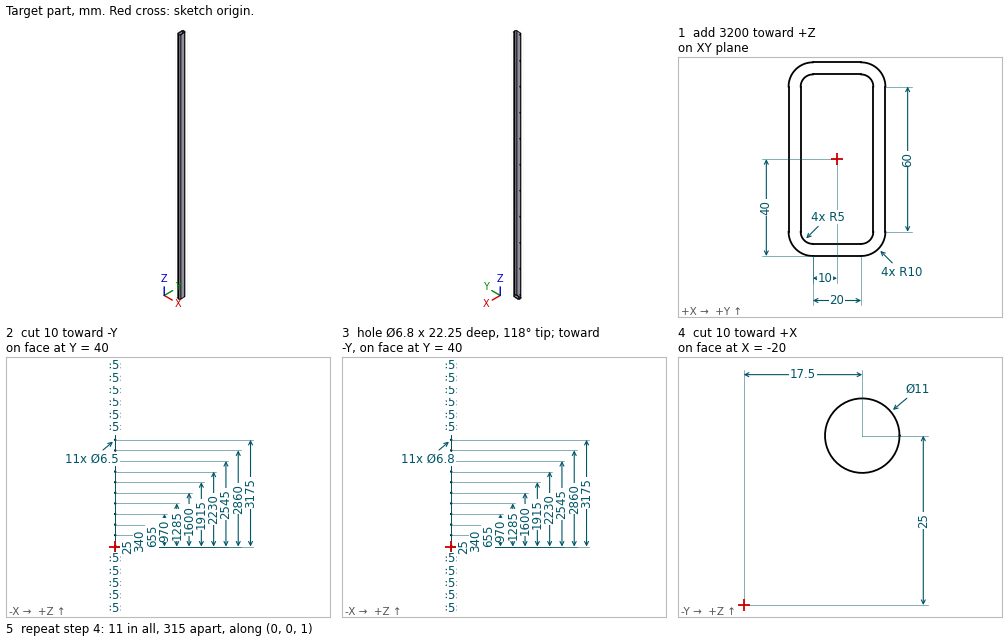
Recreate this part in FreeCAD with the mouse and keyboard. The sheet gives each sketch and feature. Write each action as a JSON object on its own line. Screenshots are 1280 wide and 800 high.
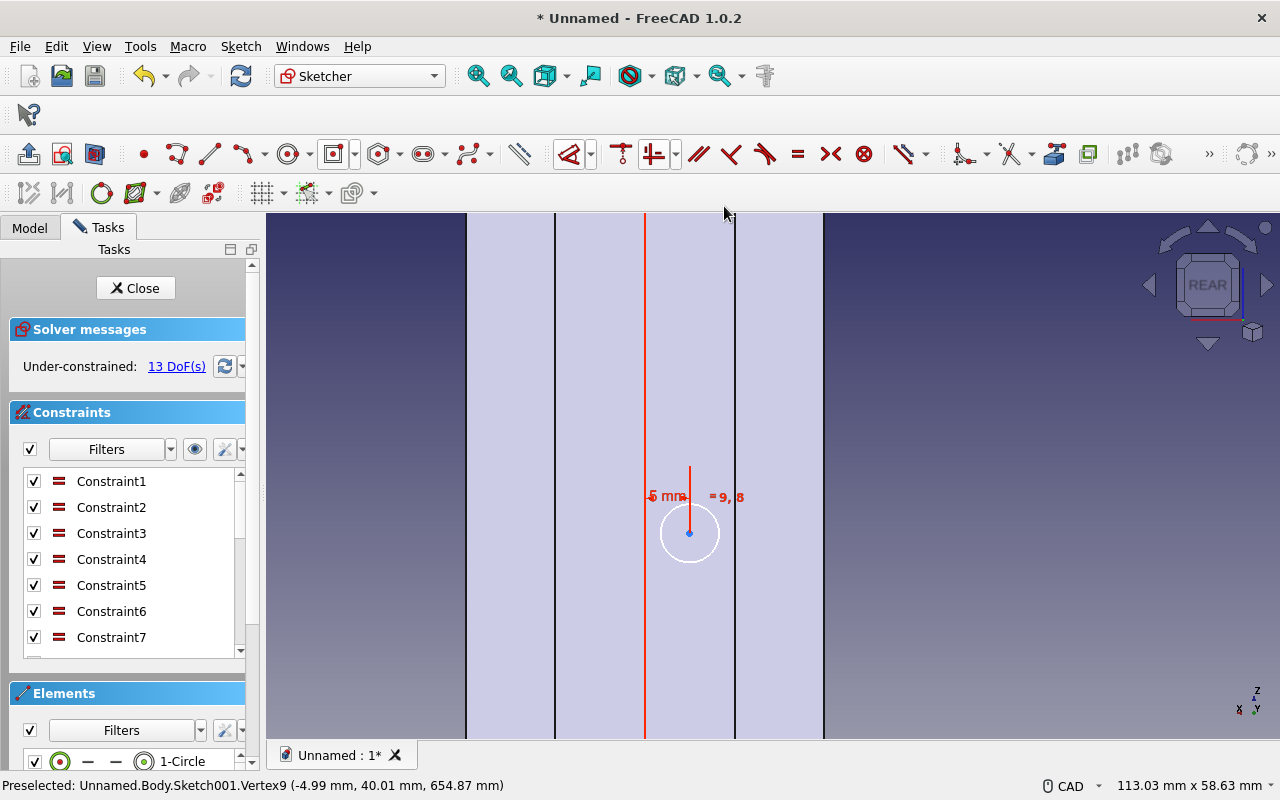
{"action": "scroll", "coordinate": [704, 476], "scroll_direction": "down", "scroll_amount": 15}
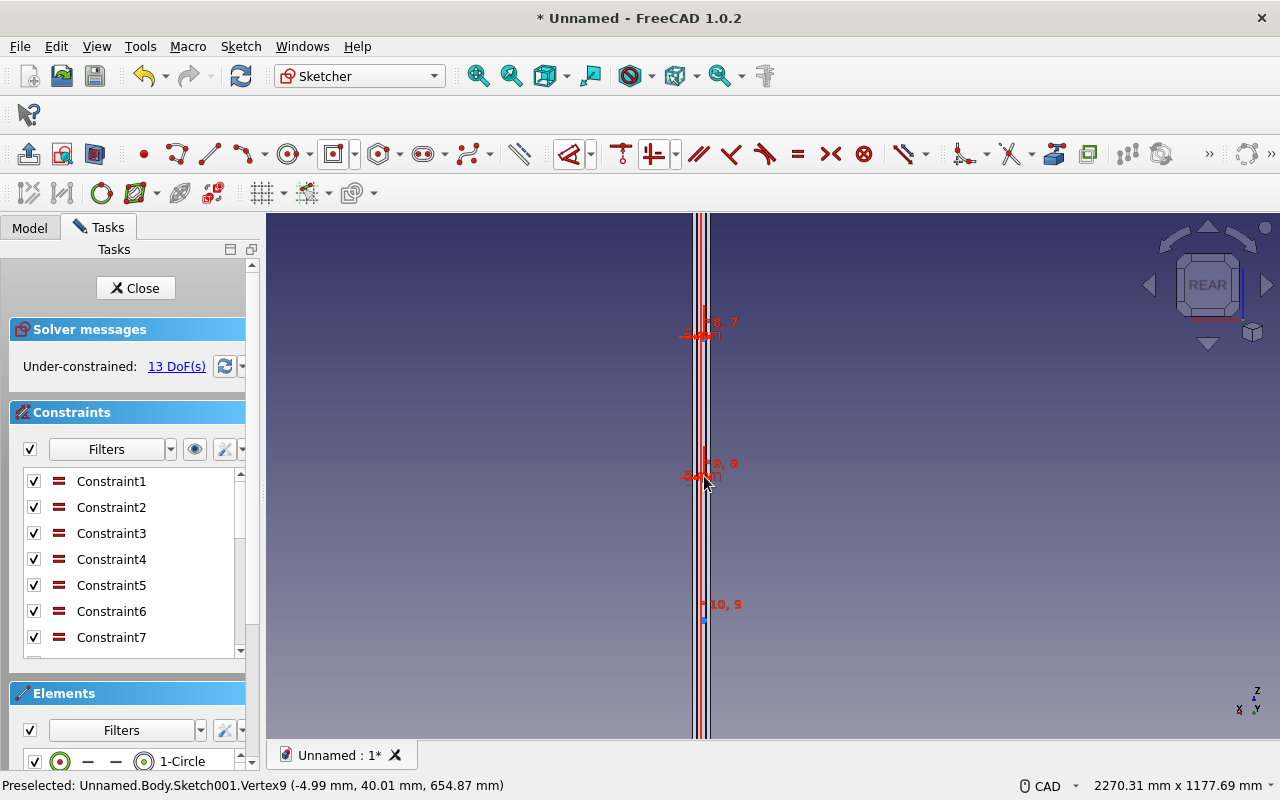
{"action": "scroll", "coordinate": [705, 611], "scroll_direction": "down", "scroll_amount": 7}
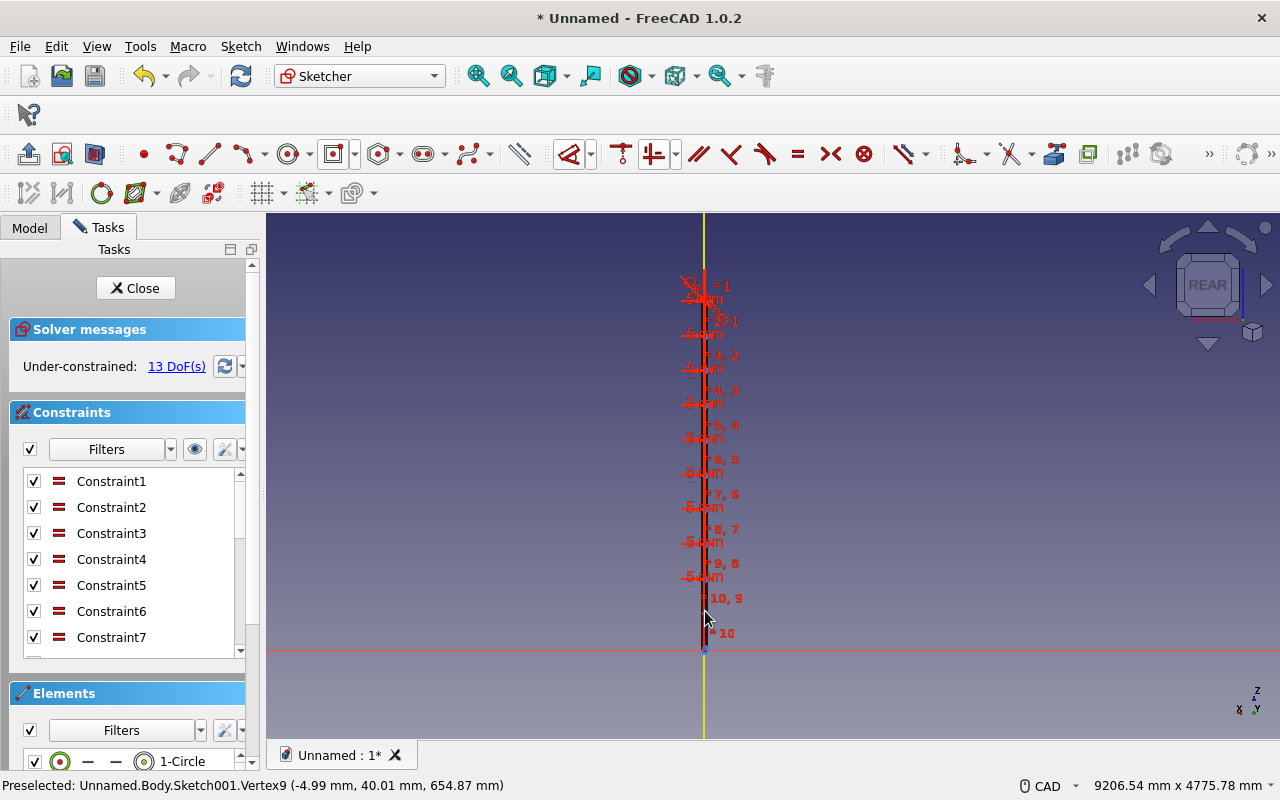
{"action": "scroll", "coordinate": [705, 614], "scroll_direction": "up", "scroll_amount": 22}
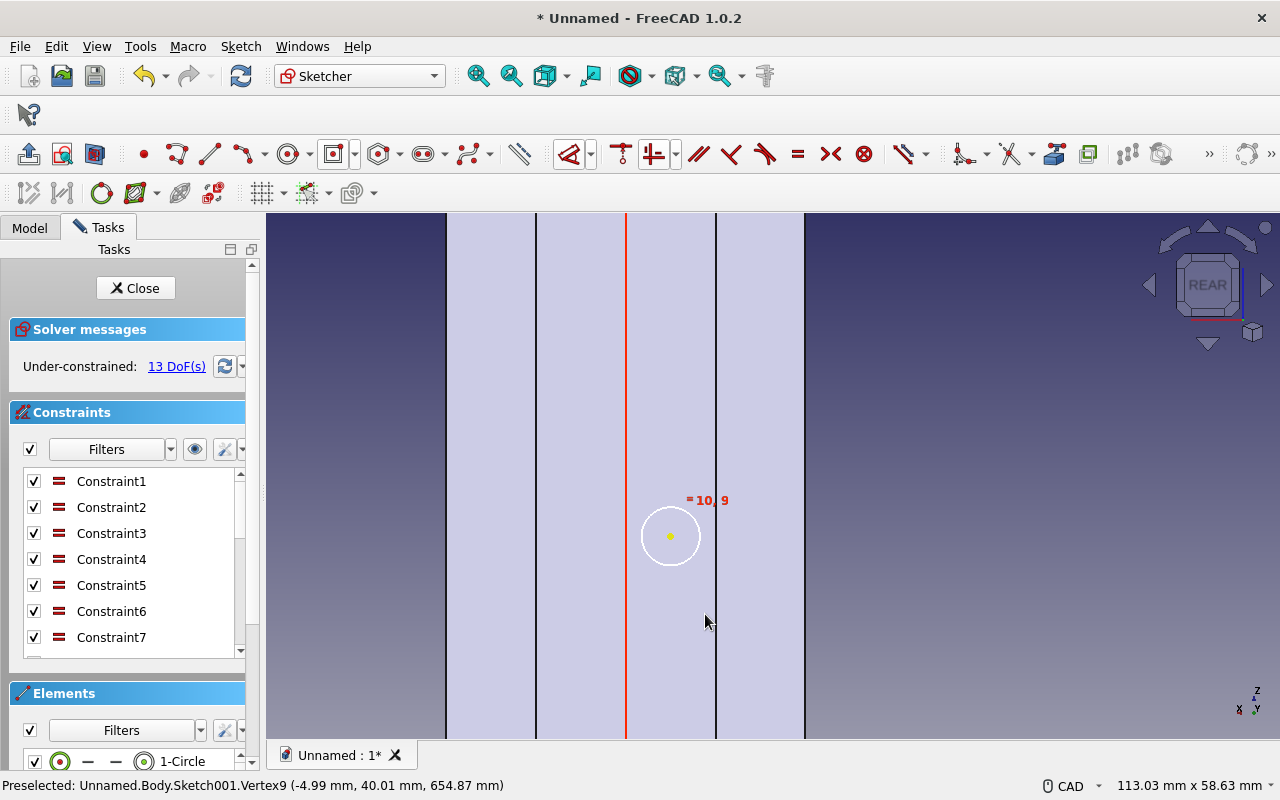
{"action": "left_click", "coordinate": [671, 536]}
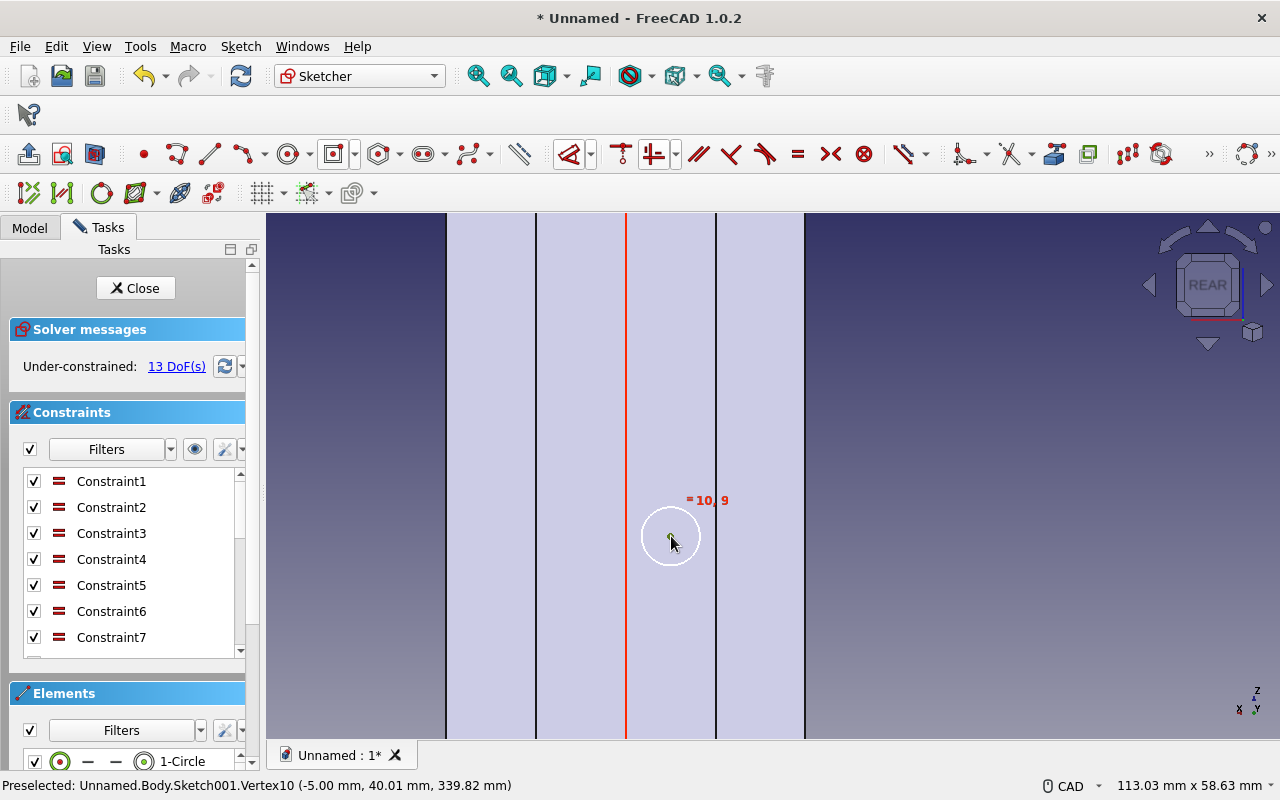
{"action": "key", "text": "l"}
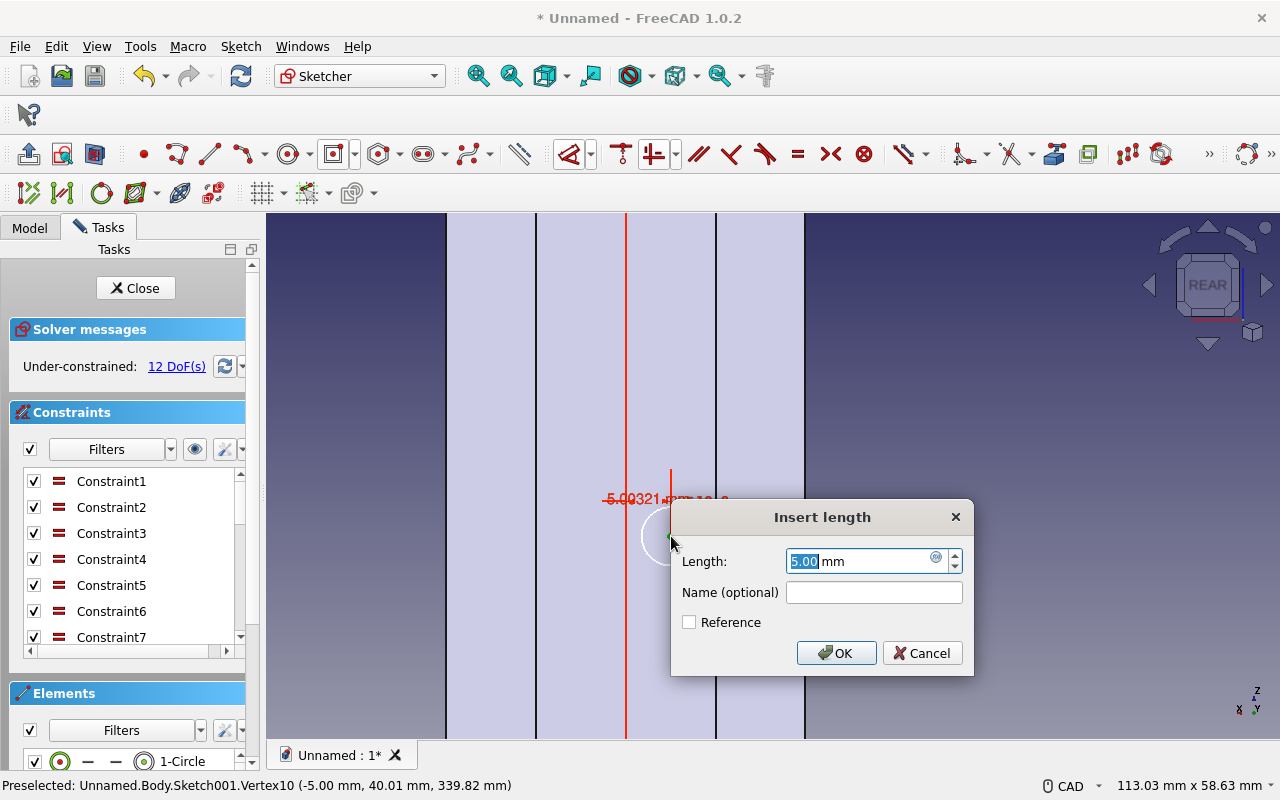
{"action": "type", "text": "5"}
{"action": "key", "text": "Return"}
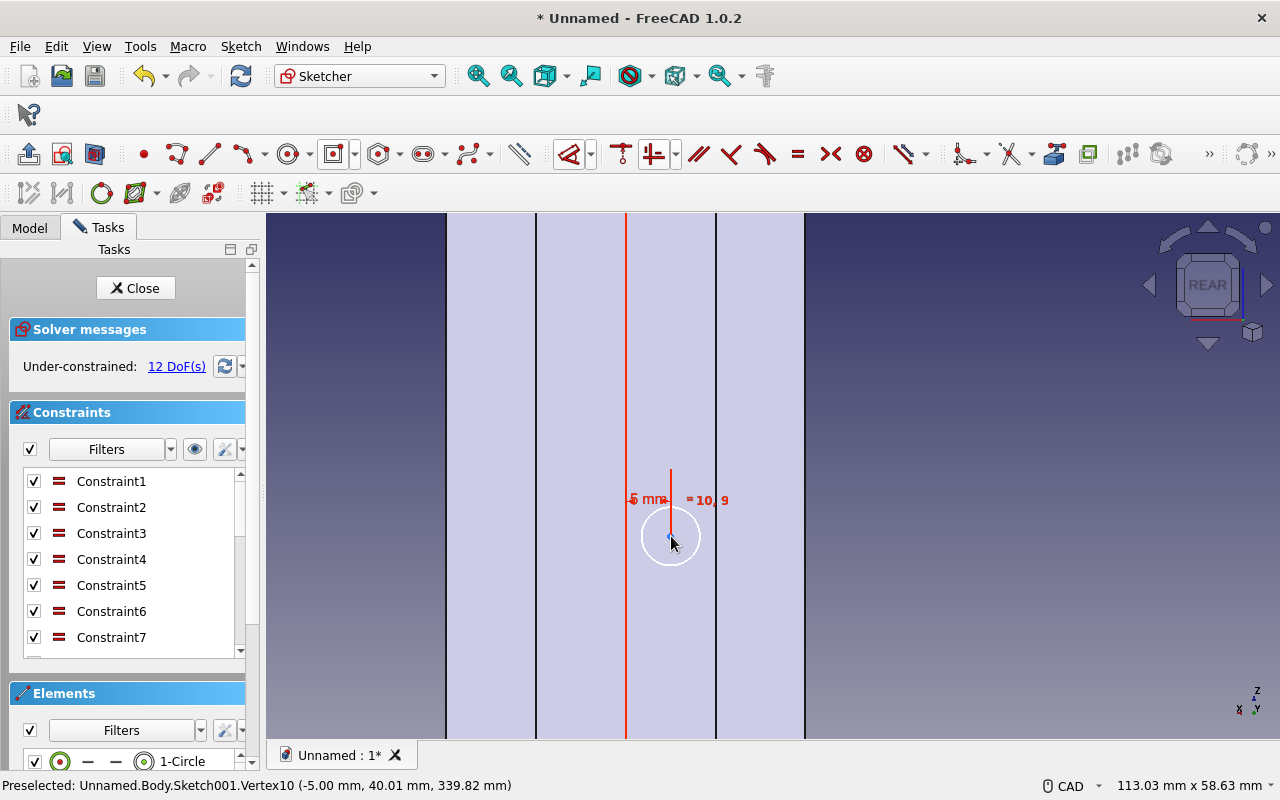
{"action": "scroll", "coordinate": [704, 476], "scroll_direction": "down", "scroll_amount": 15}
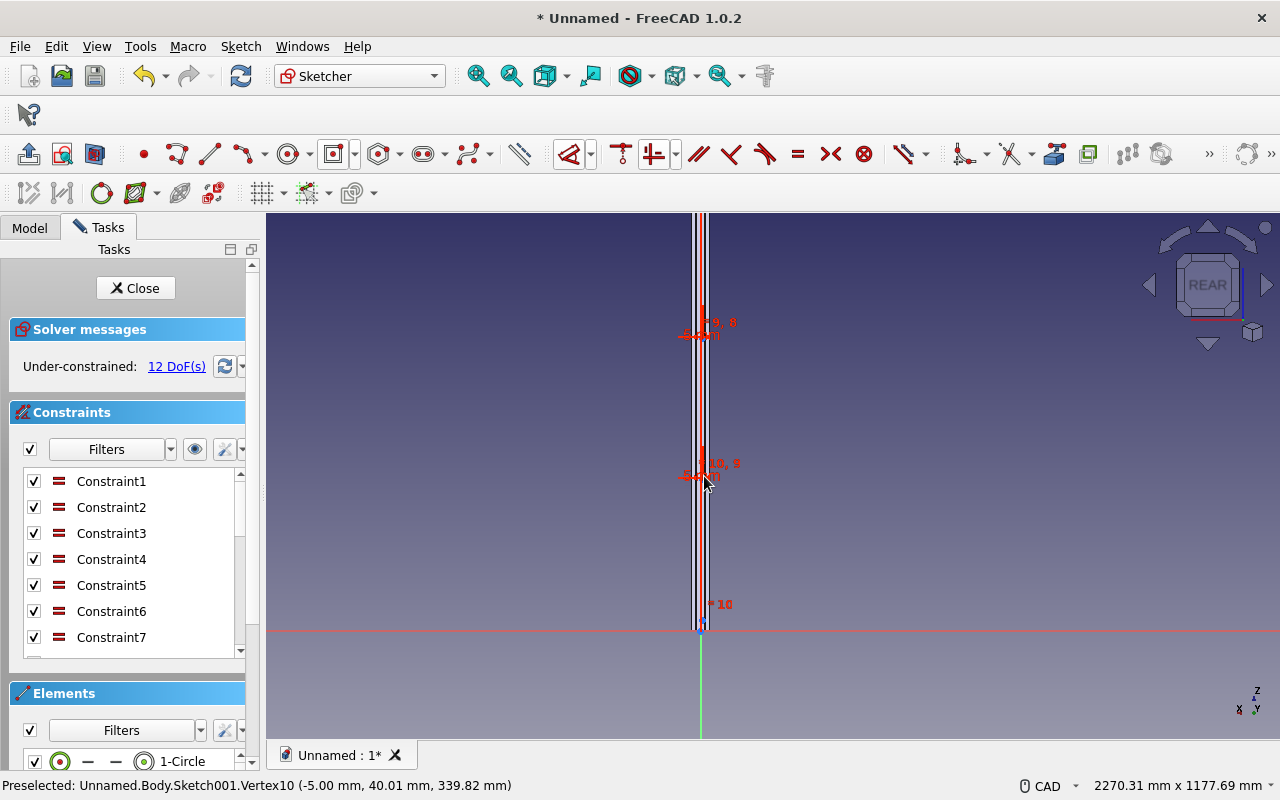
{"action": "scroll", "coordinate": [705, 657], "scroll_direction": "down", "scroll_amount": 7}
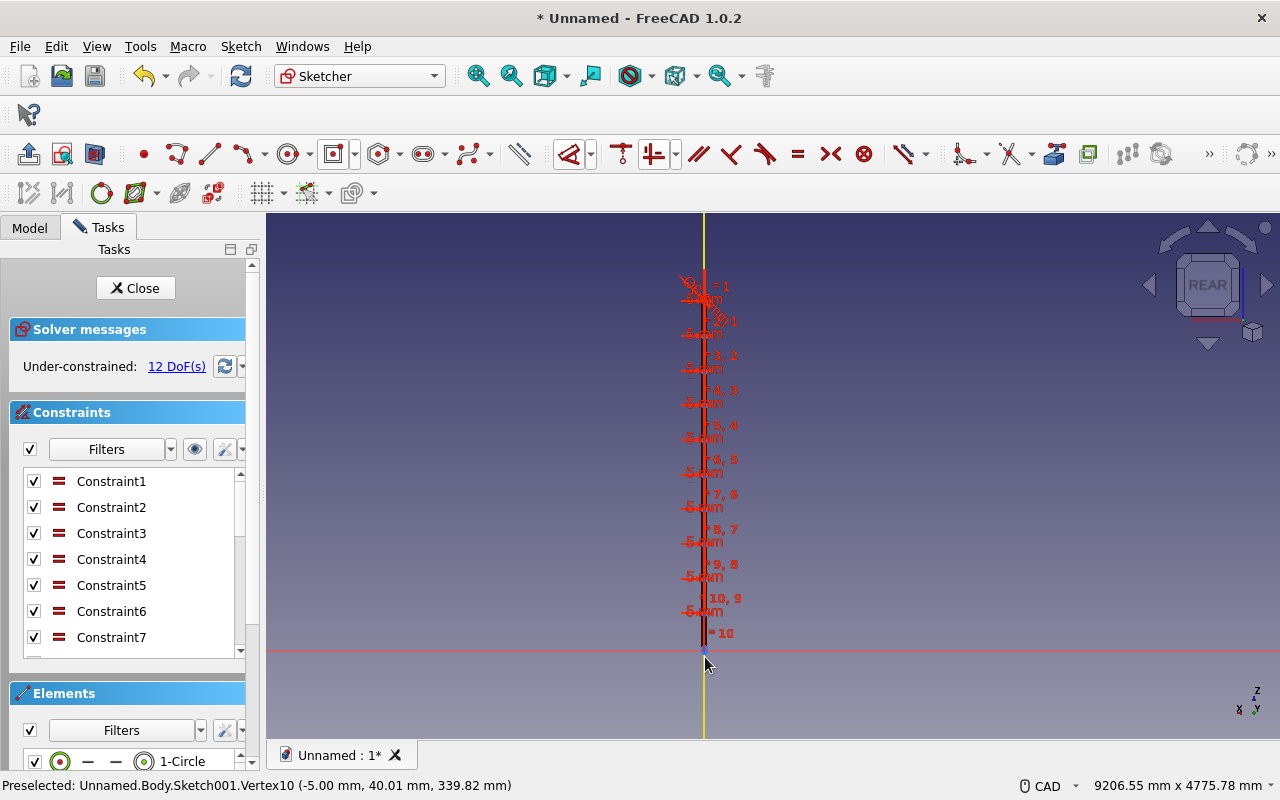
{"action": "scroll", "coordinate": [705, 649], "scroll_direction": "up", "scroll_amount": 22}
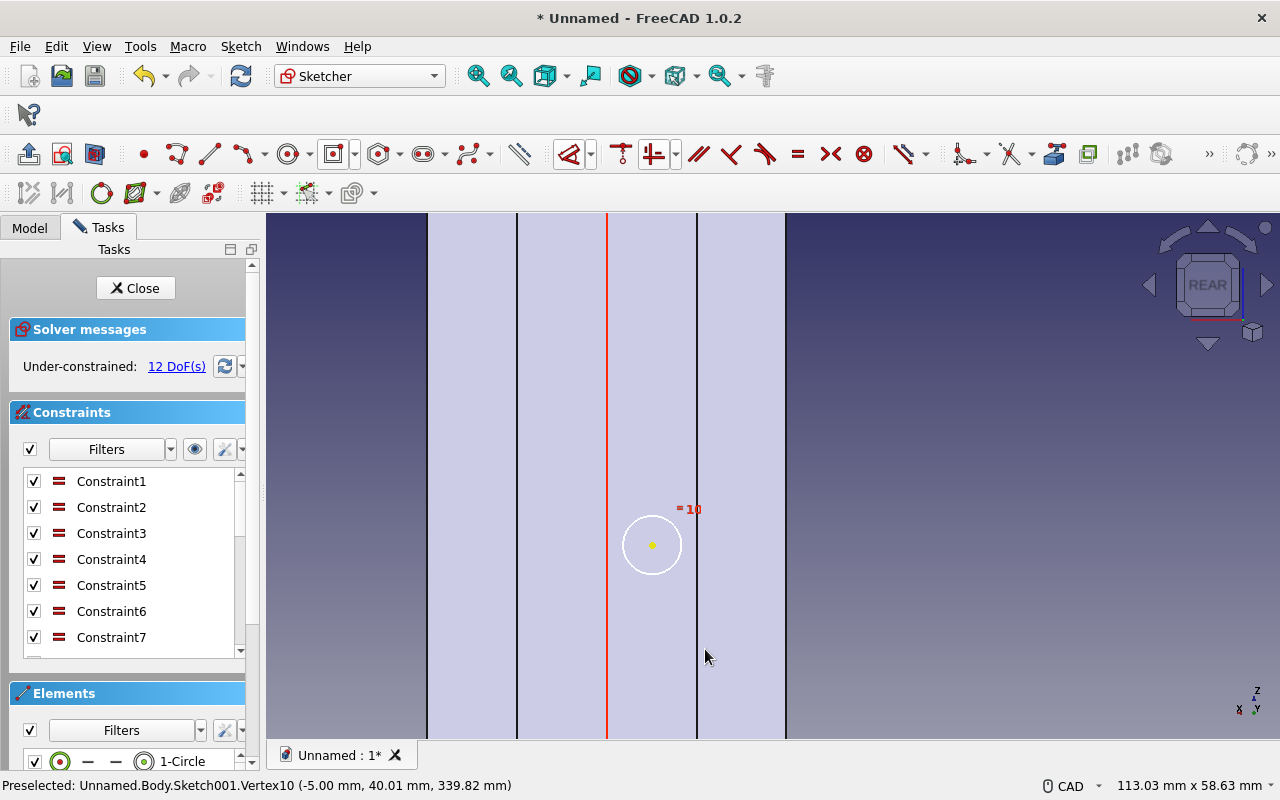
{"action": "left_click", "coordinate": [652, 545]}